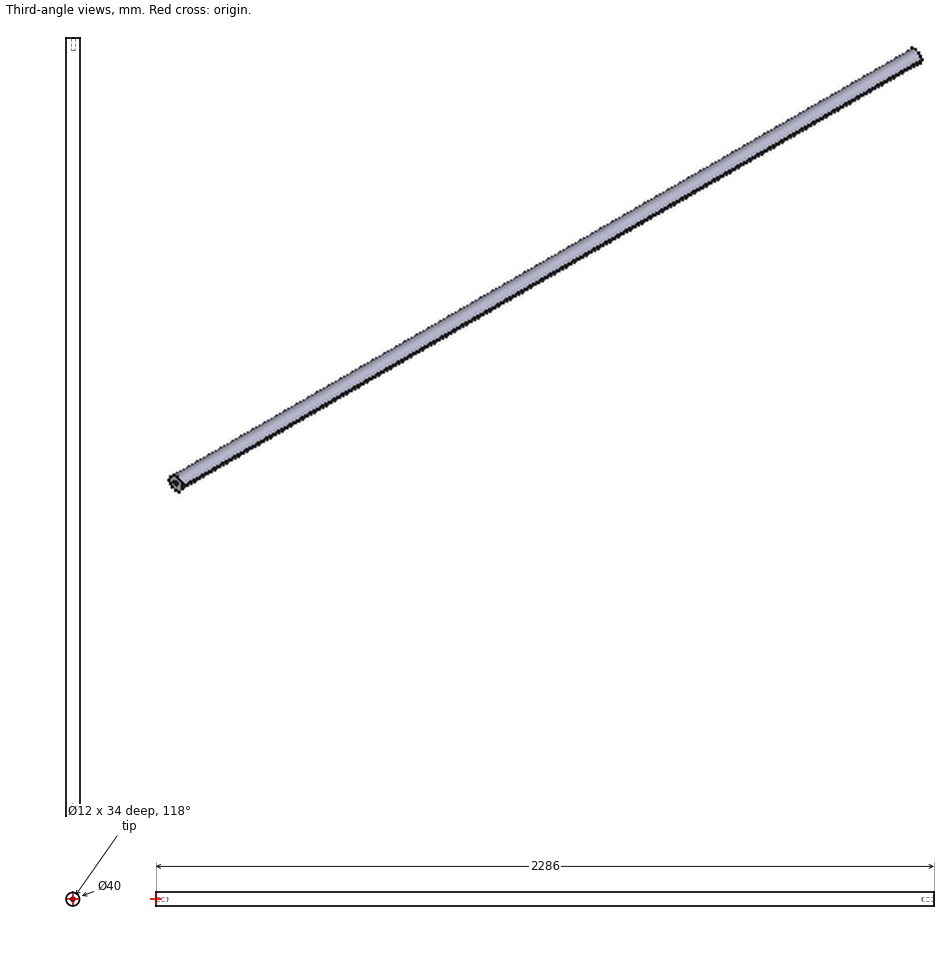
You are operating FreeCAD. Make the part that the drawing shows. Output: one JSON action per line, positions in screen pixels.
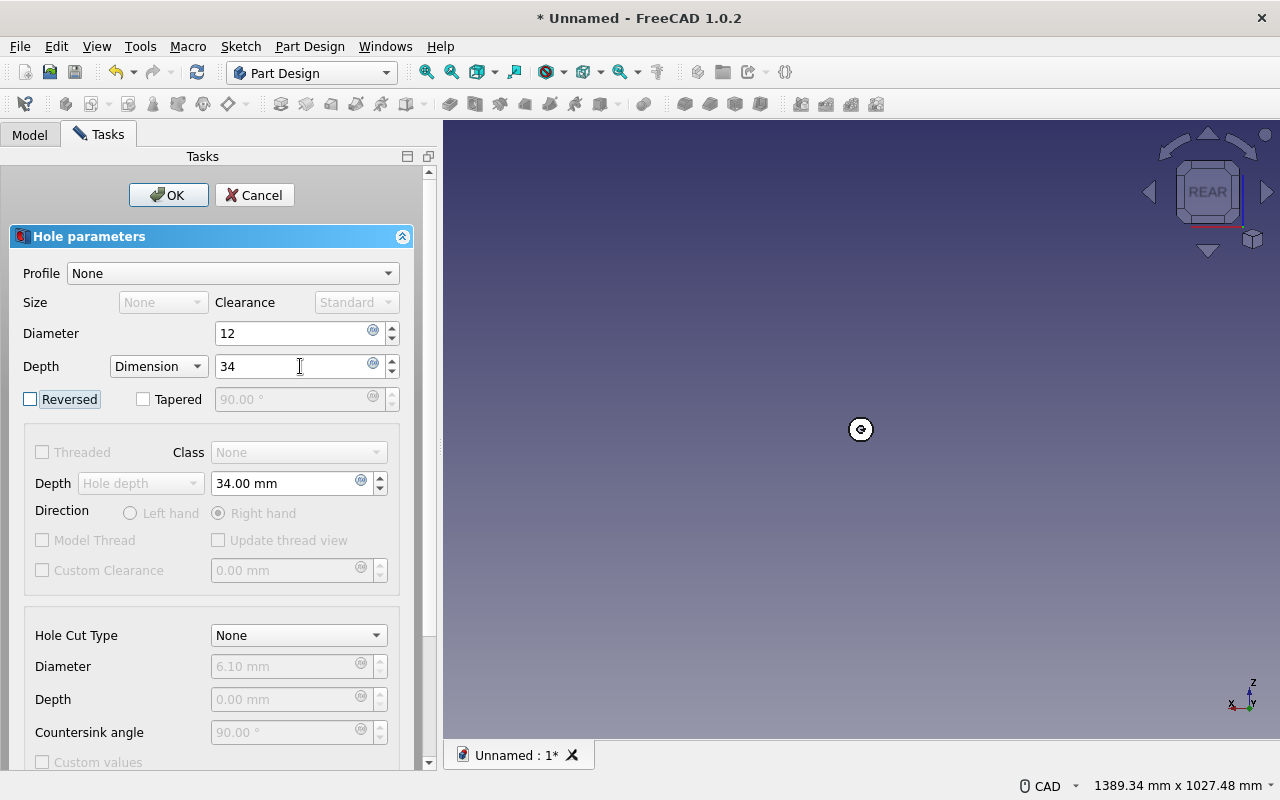
{"action": "left_click", "coordinate": [169, 195]}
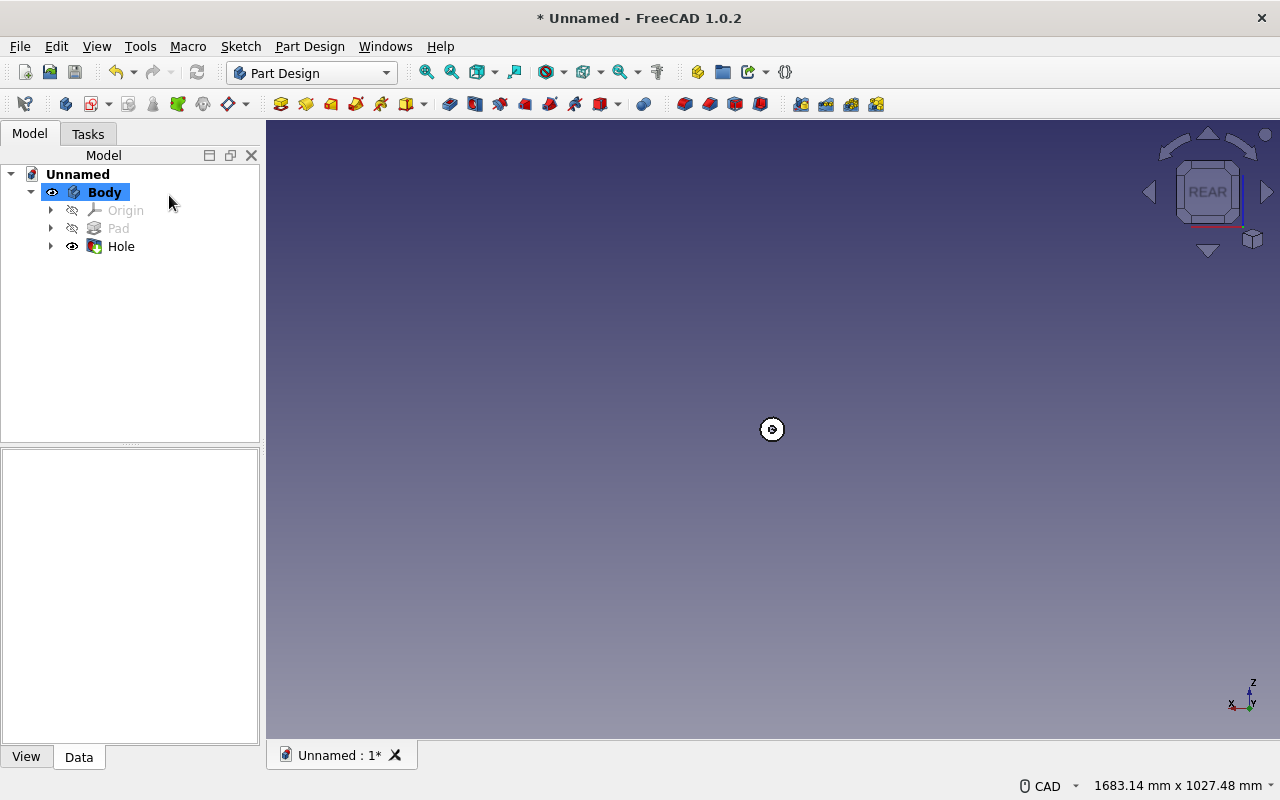
{"action": "left_click", "coordinate": [427, 72]}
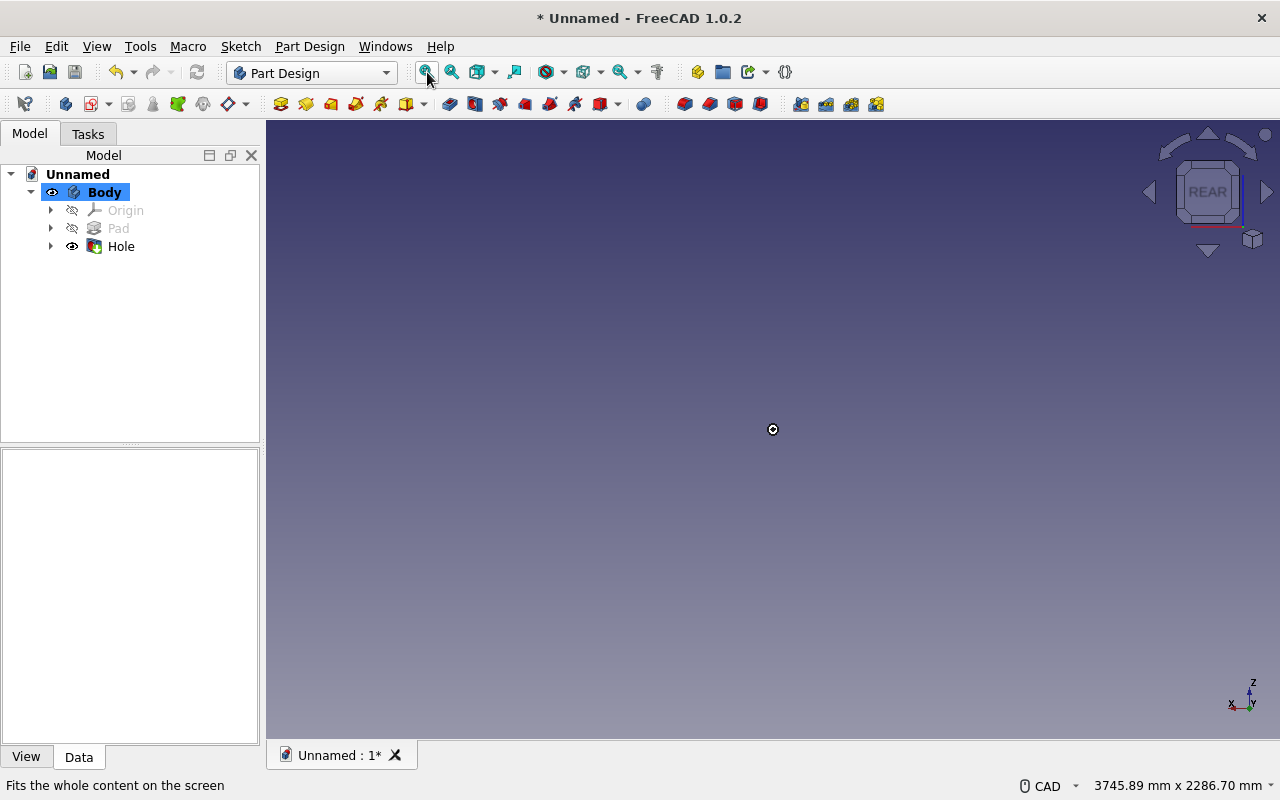
{"action": "left_click", "coordinate": [90, 104]}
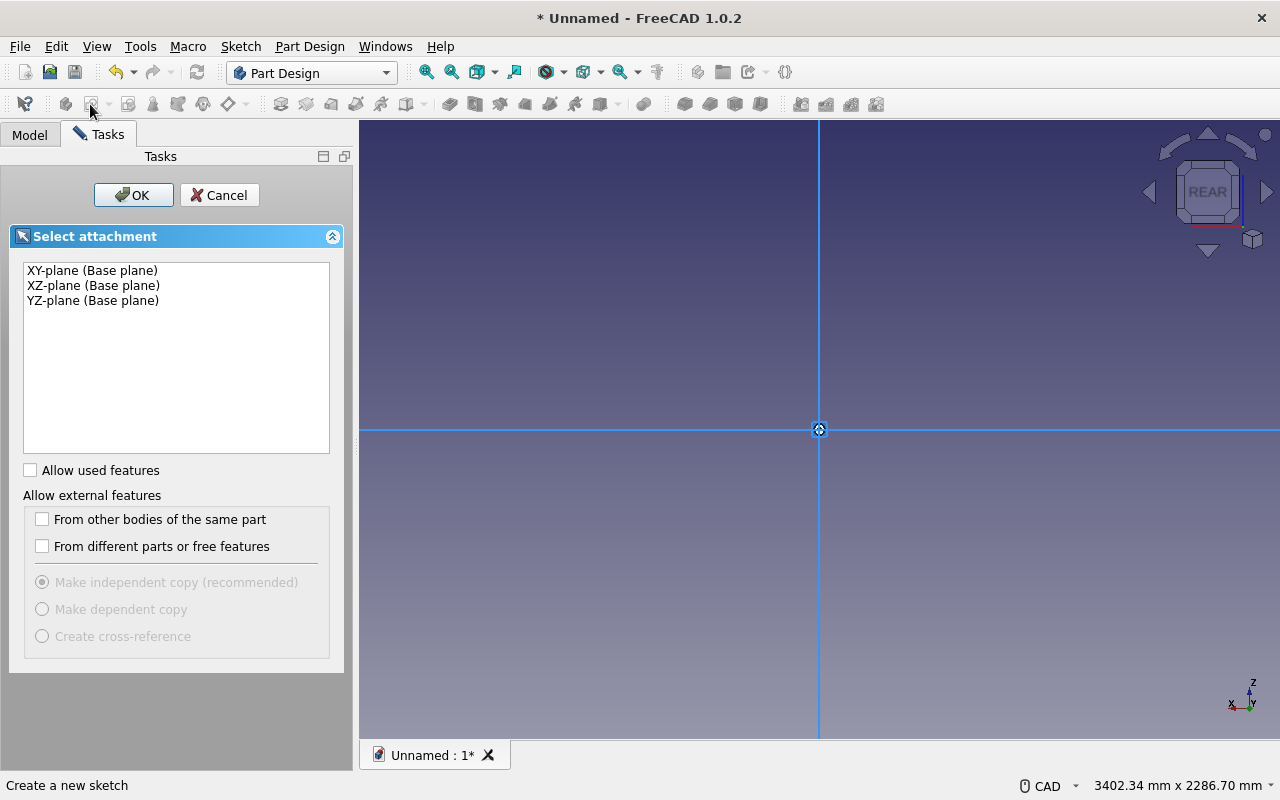
{"action": "left_click", "coordinate": [84, 286]}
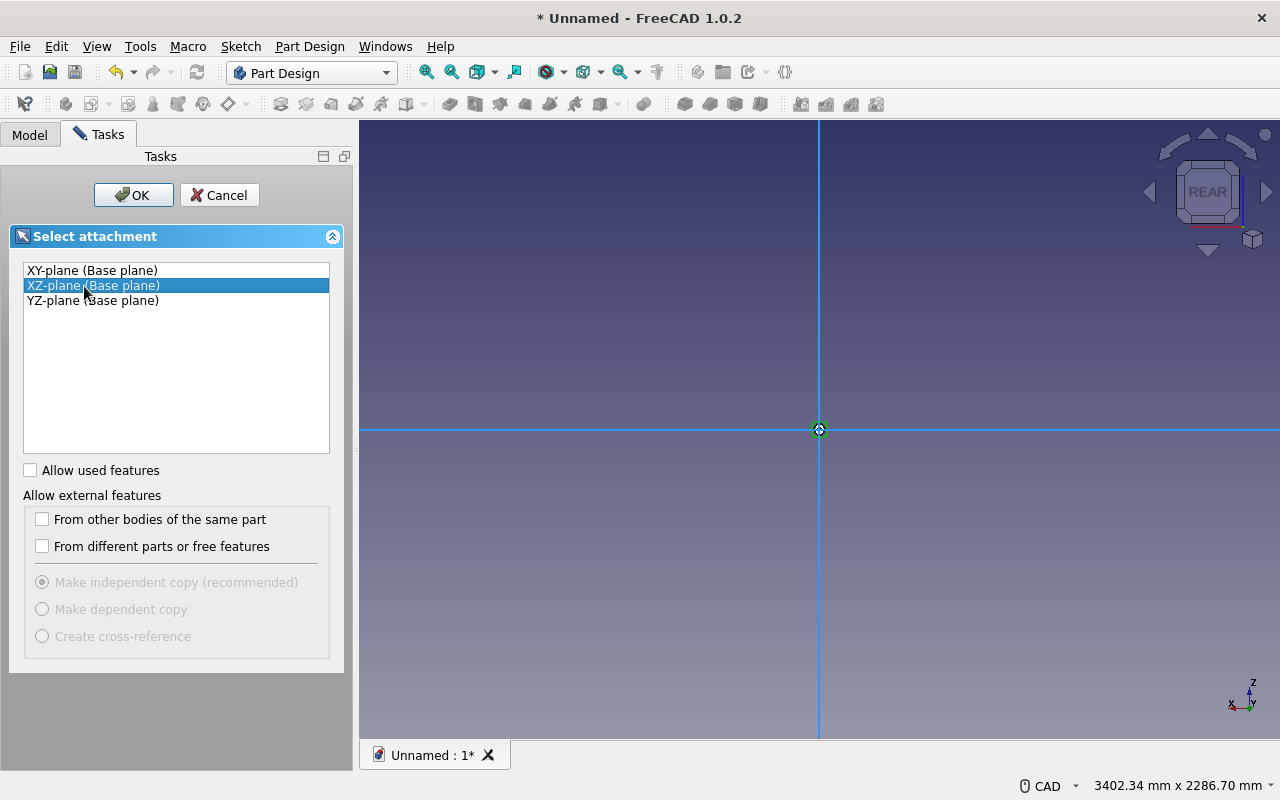
{"action": "left_click", "coordinate": [134, 195]}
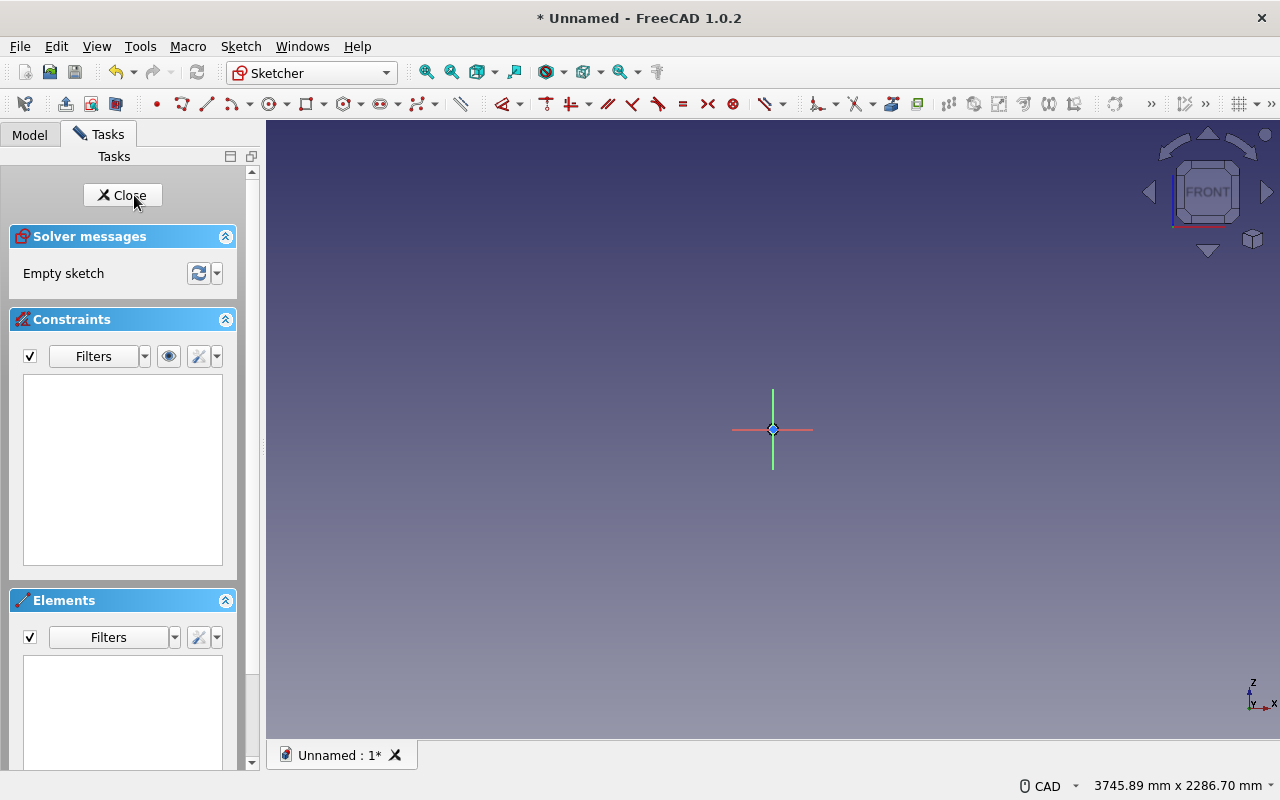
{"action": "scroll", "coordinate": [777, 430], "scroll_direction": "up", "scroll_amount": 15}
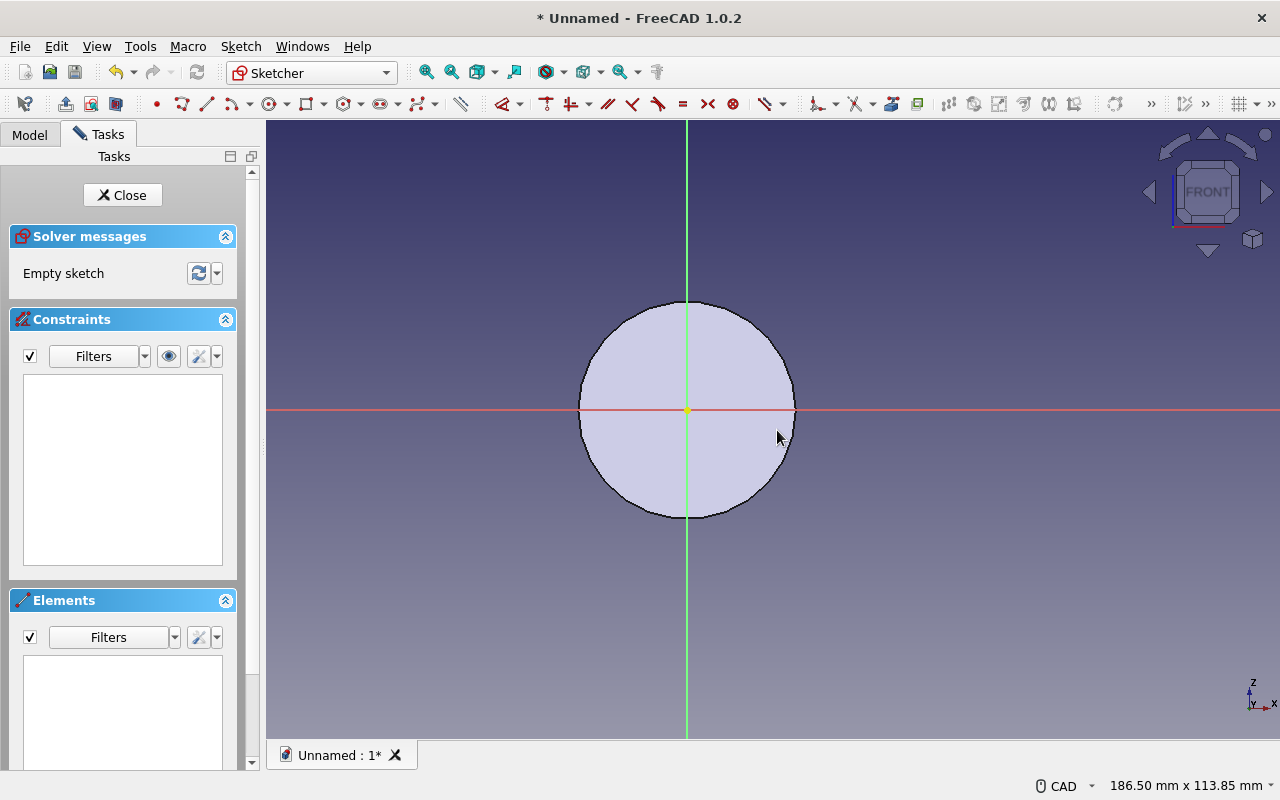
{"action": "scroll", "coordinate": [684, 407], "scroll_direction": "up", "scroll_amount": 9}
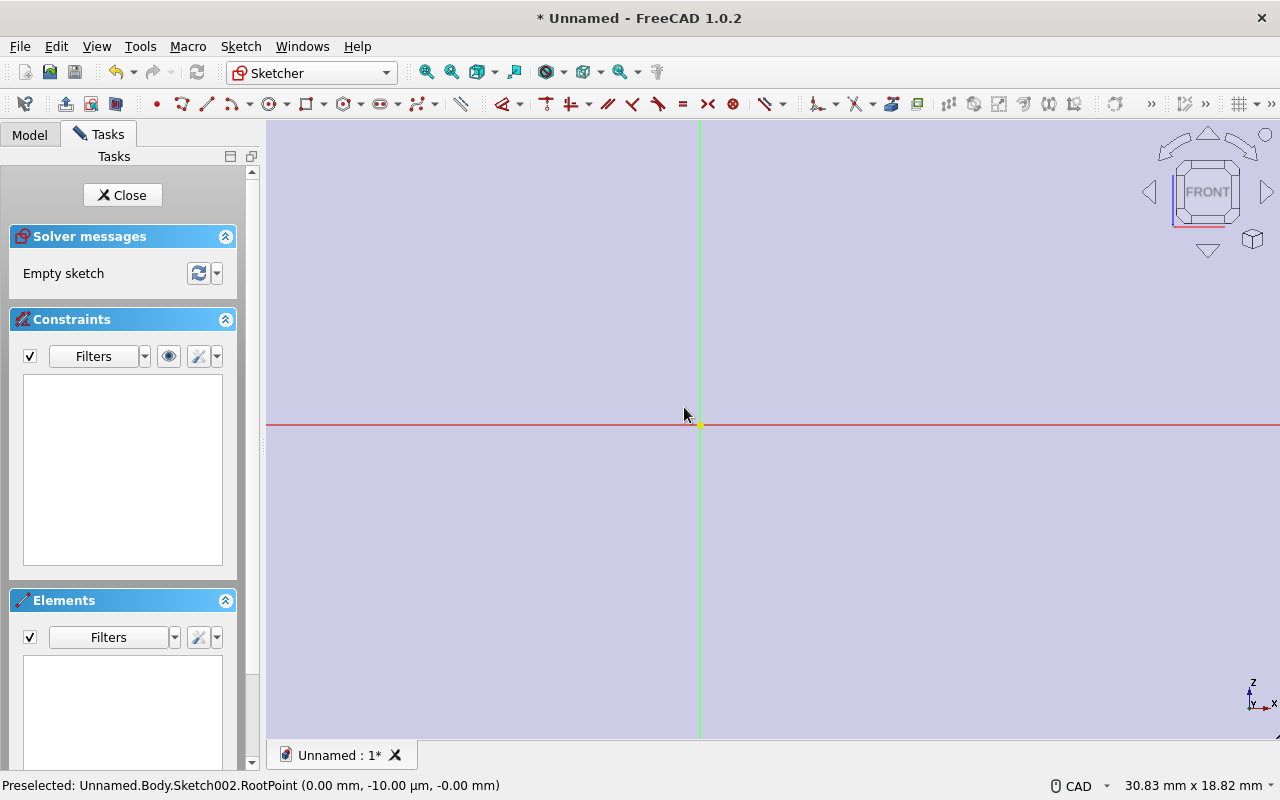
{"action": "left_click", "coordinate": [268, 104]}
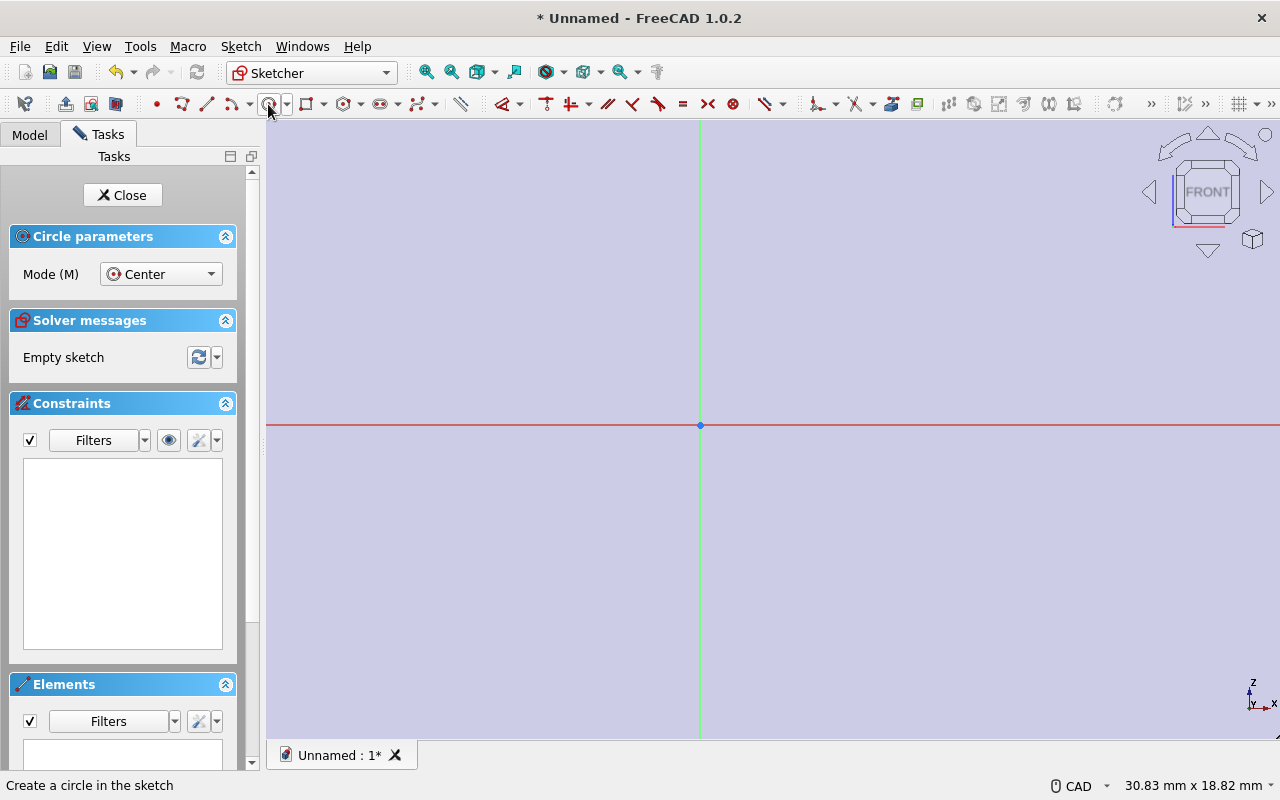
{"action": "left_click", "coordinate": [700, 425]}
{"action": "mouse_move", "coordinate": [840, 286]}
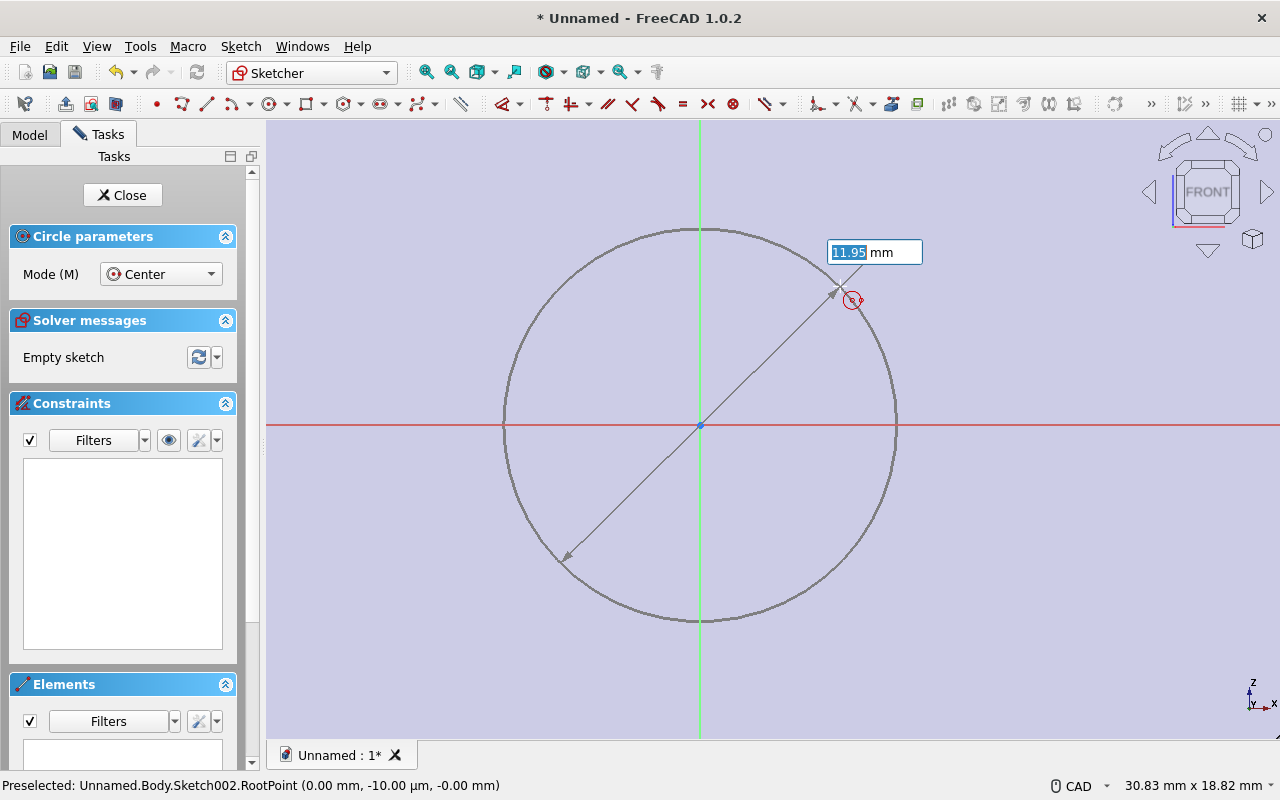
{"action": "type", "text": "12"}
{"action": "key", "text": "Return"}
{"action": "key", "text": "Escape"}